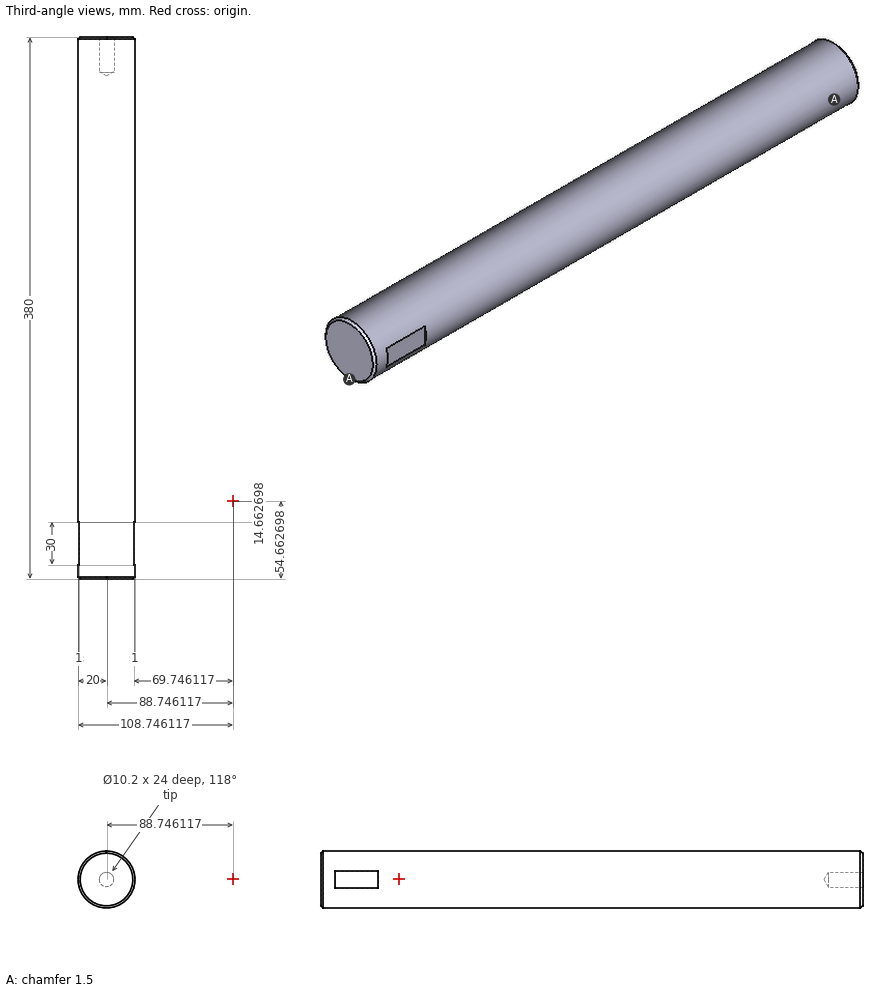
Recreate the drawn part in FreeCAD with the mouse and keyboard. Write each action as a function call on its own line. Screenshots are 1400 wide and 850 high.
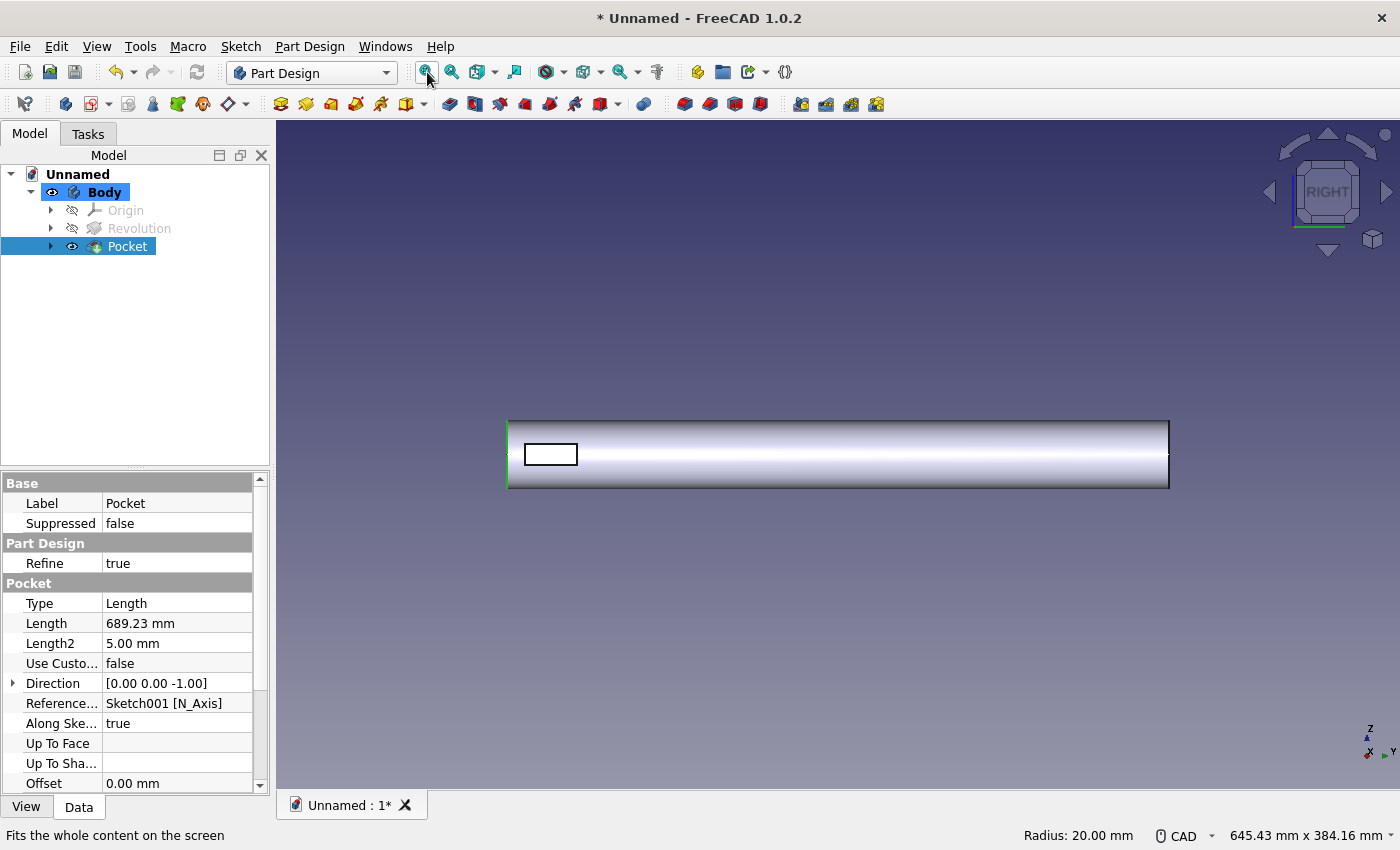
click(1169, 453, ctrl)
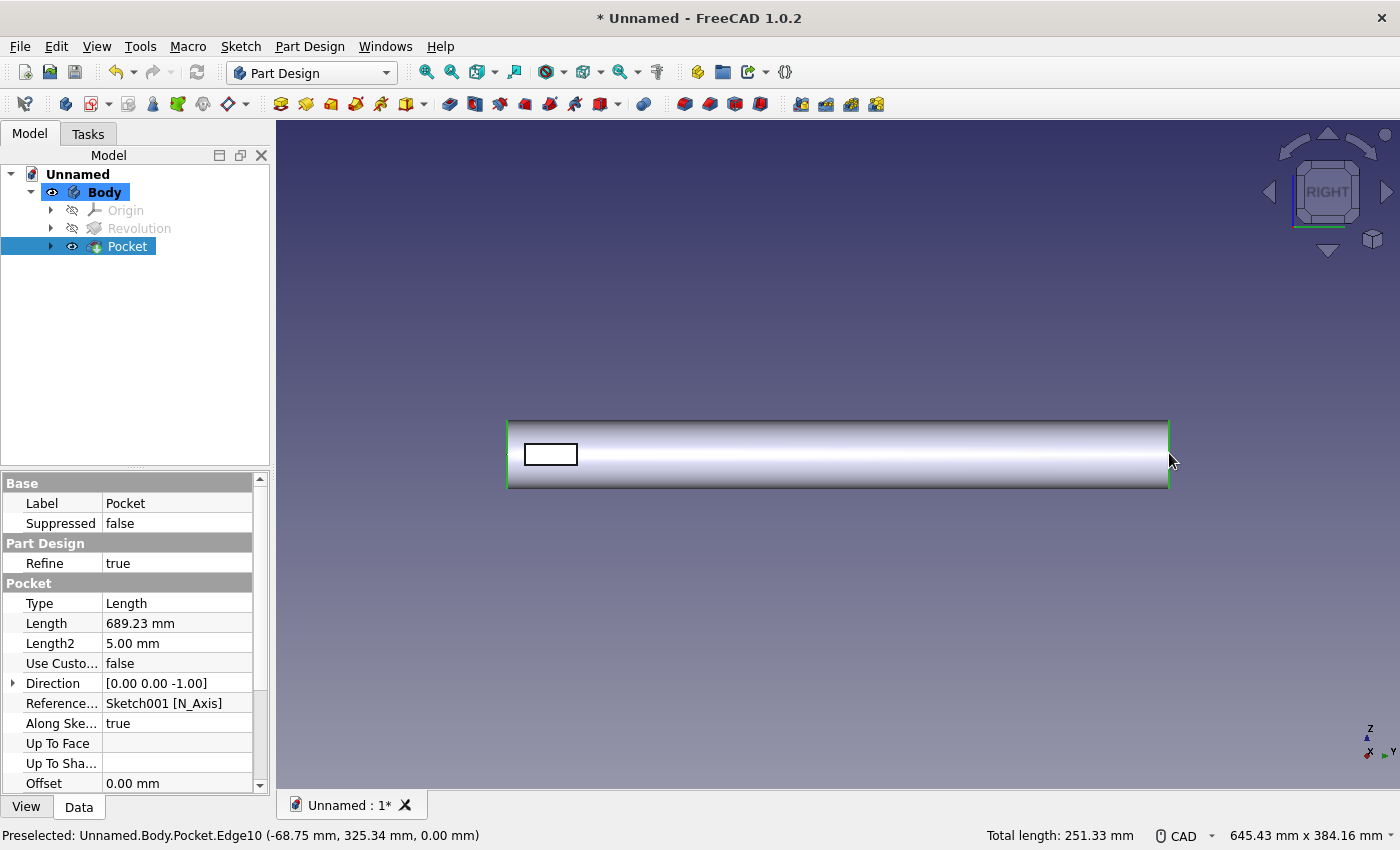
click(710, 104)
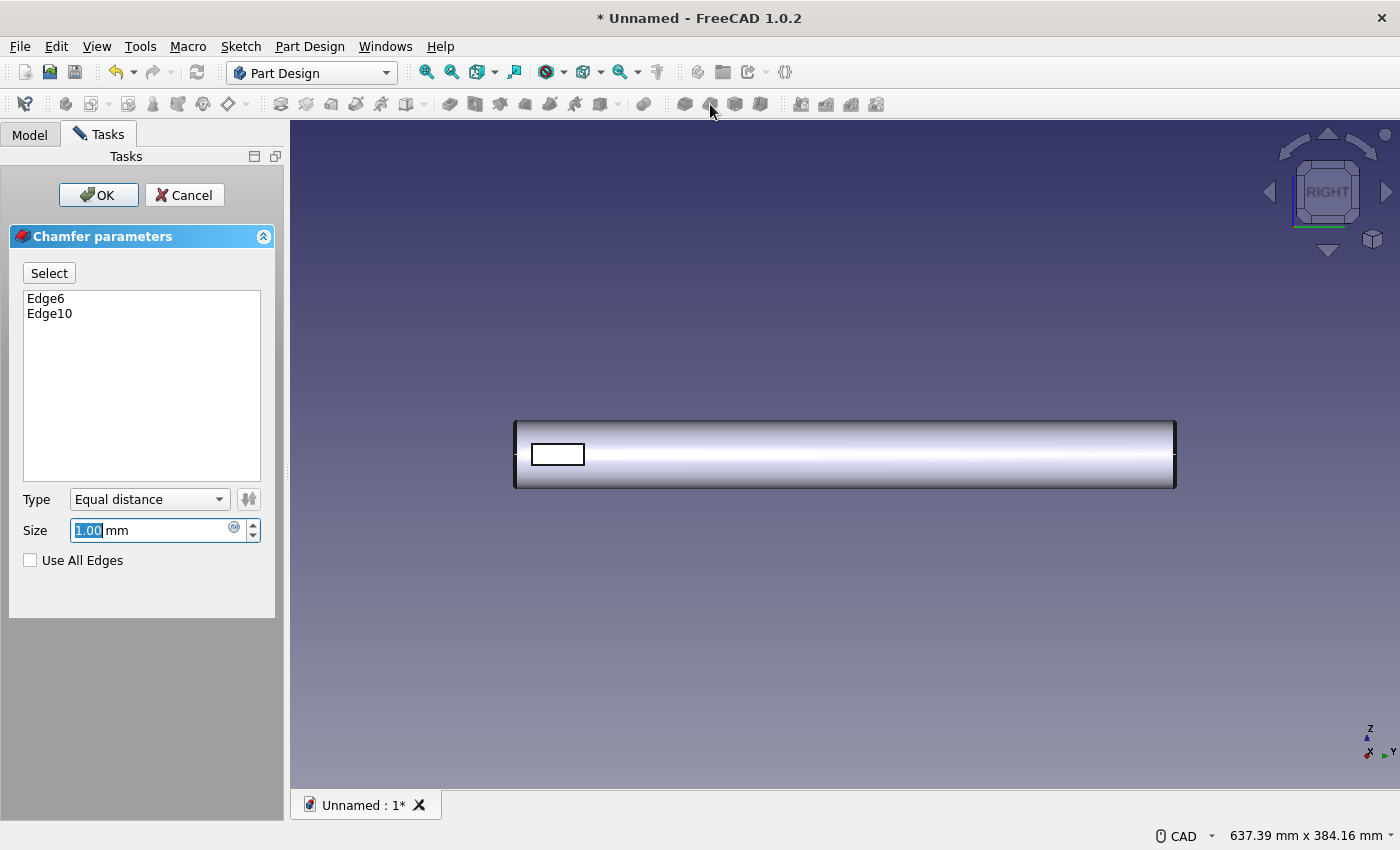
text(1.5)
key(Tab)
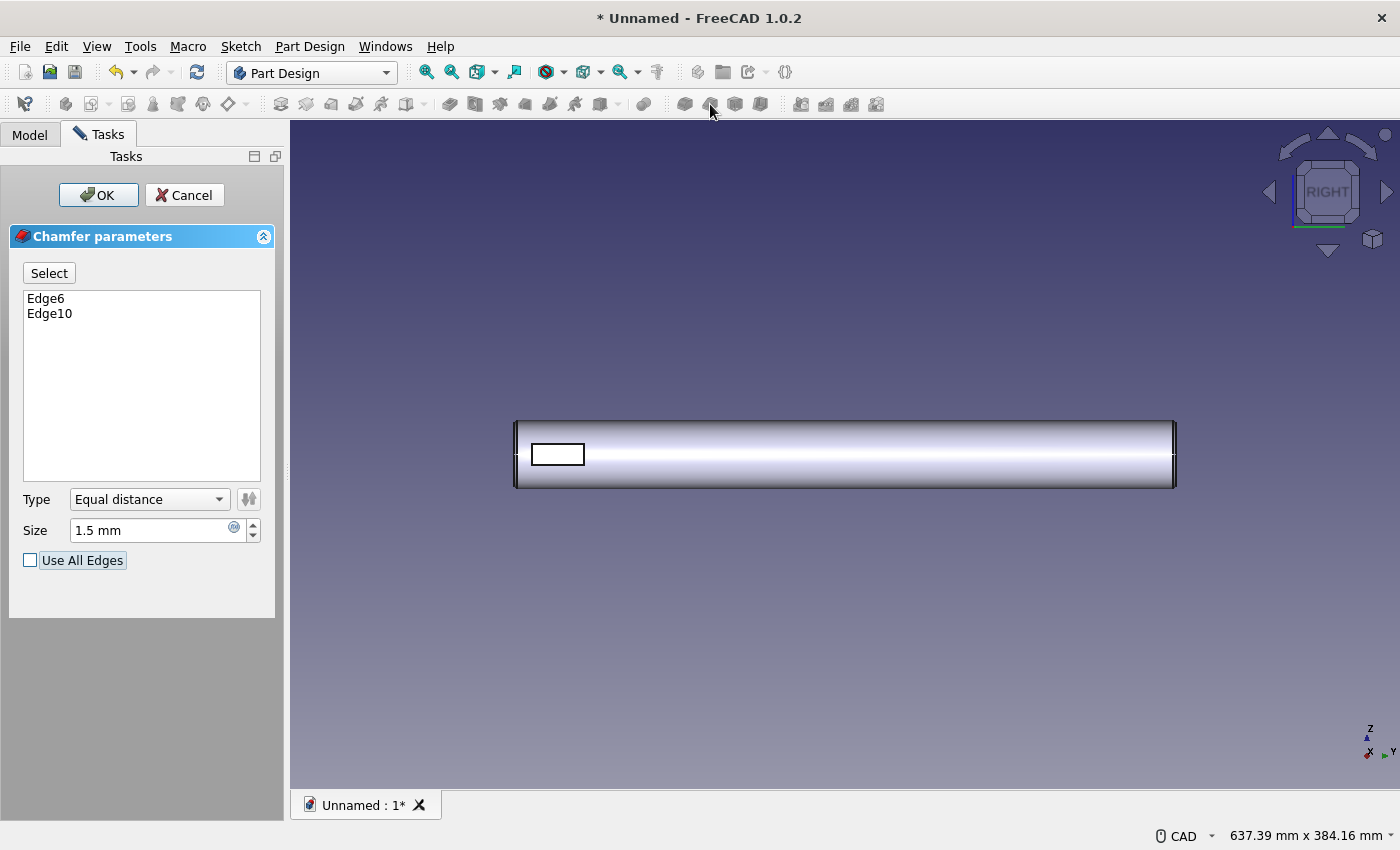
click(99, 195)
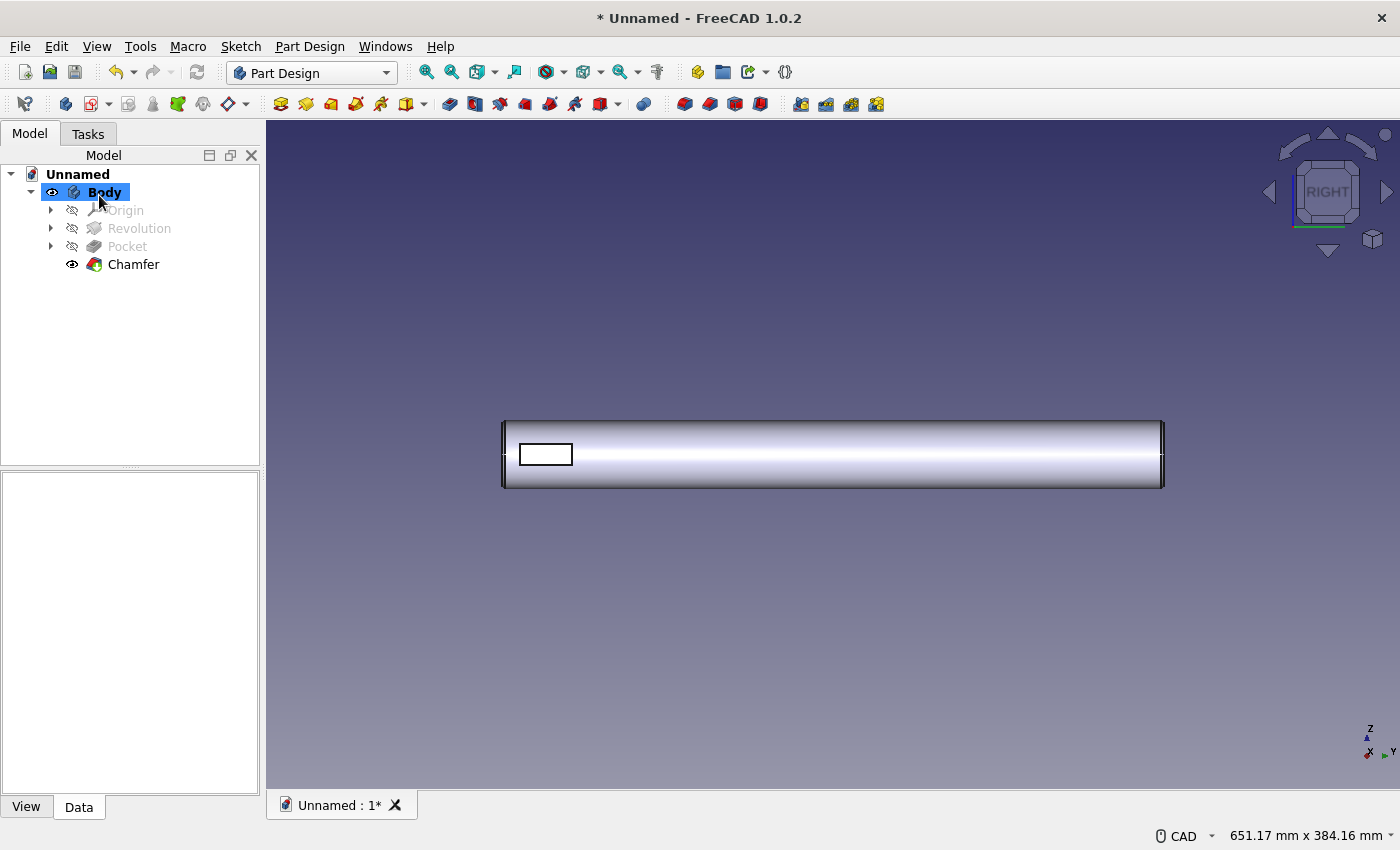
key(4)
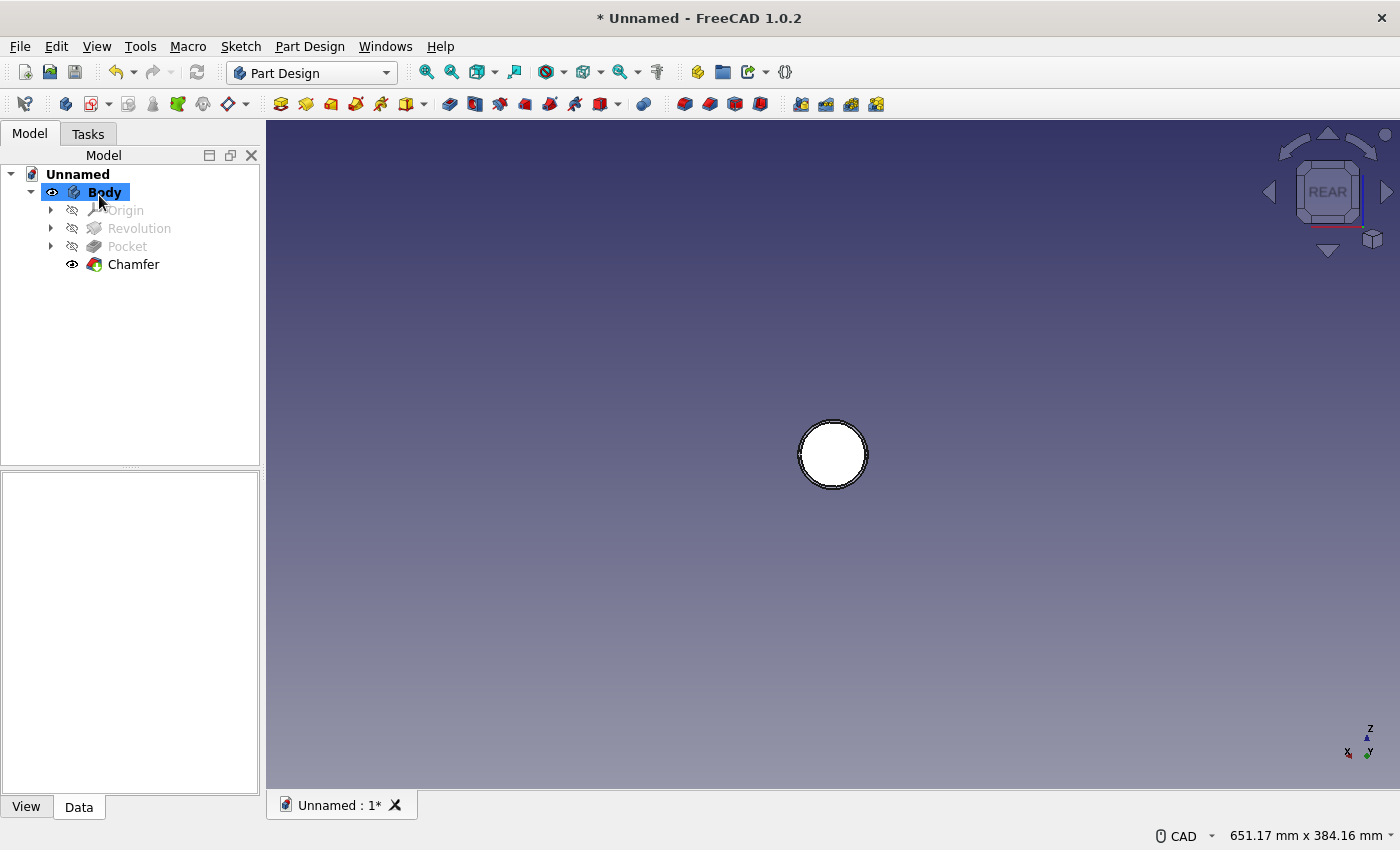
click(427, 72)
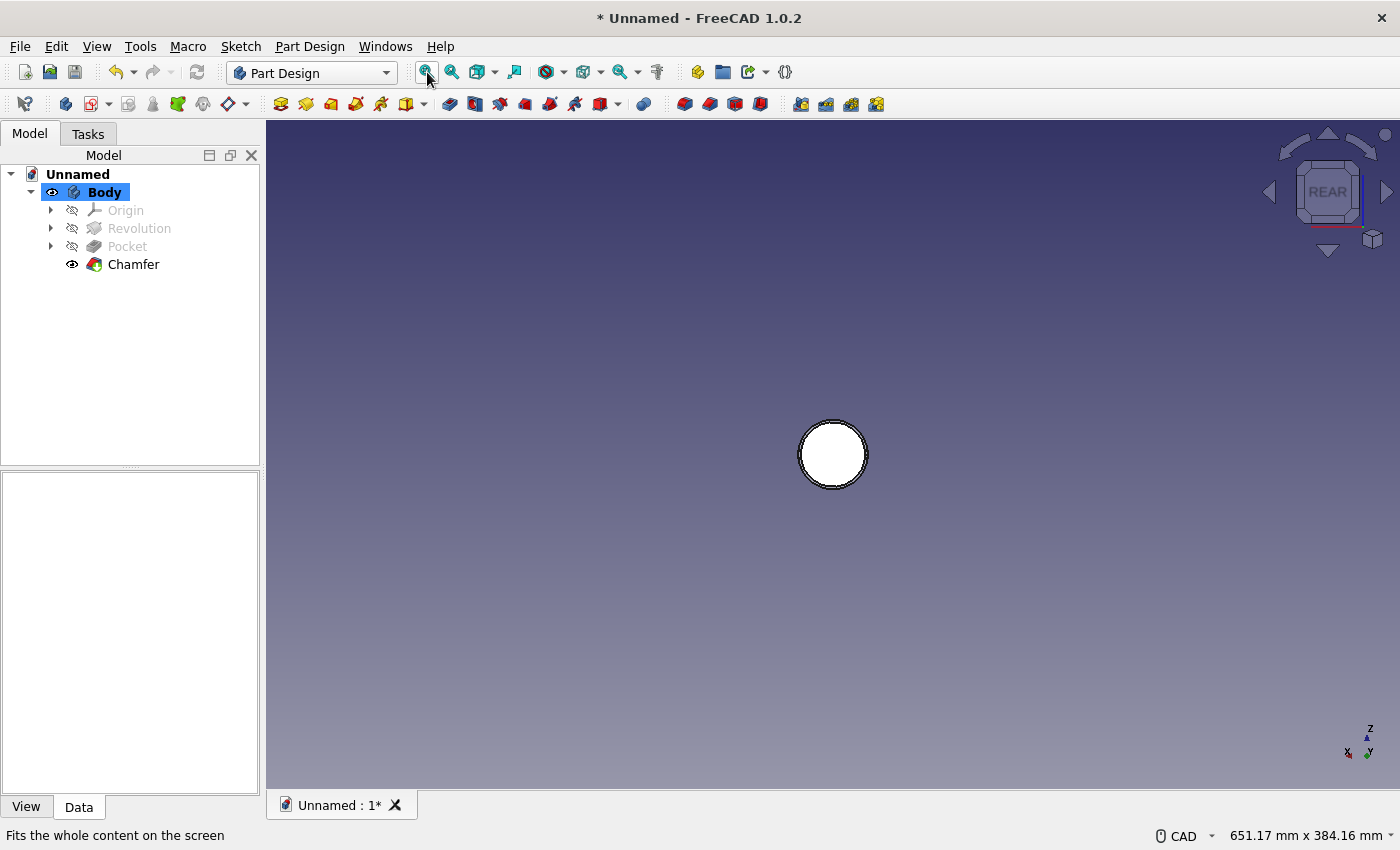
click(833, 454)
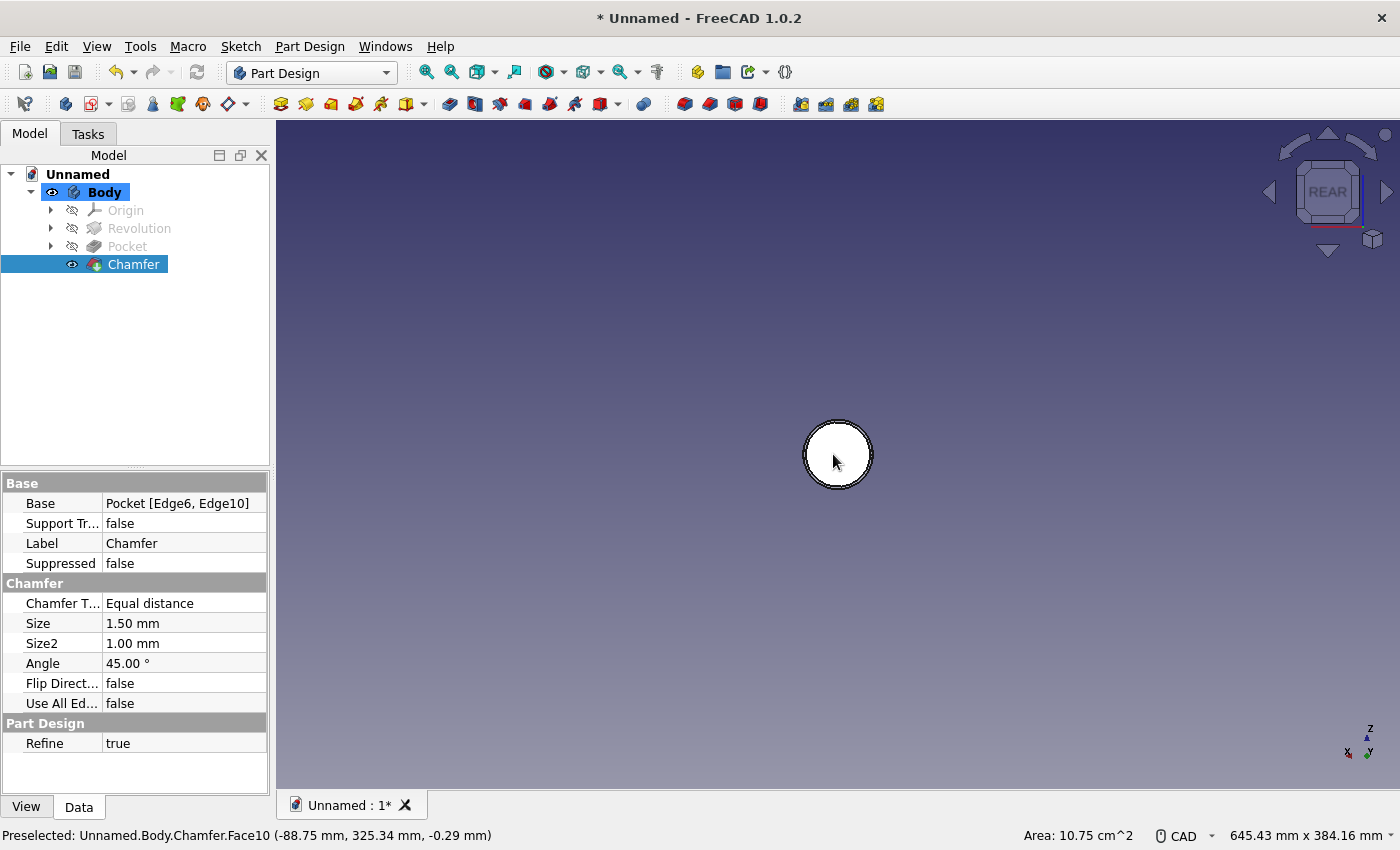
click(90, 104)